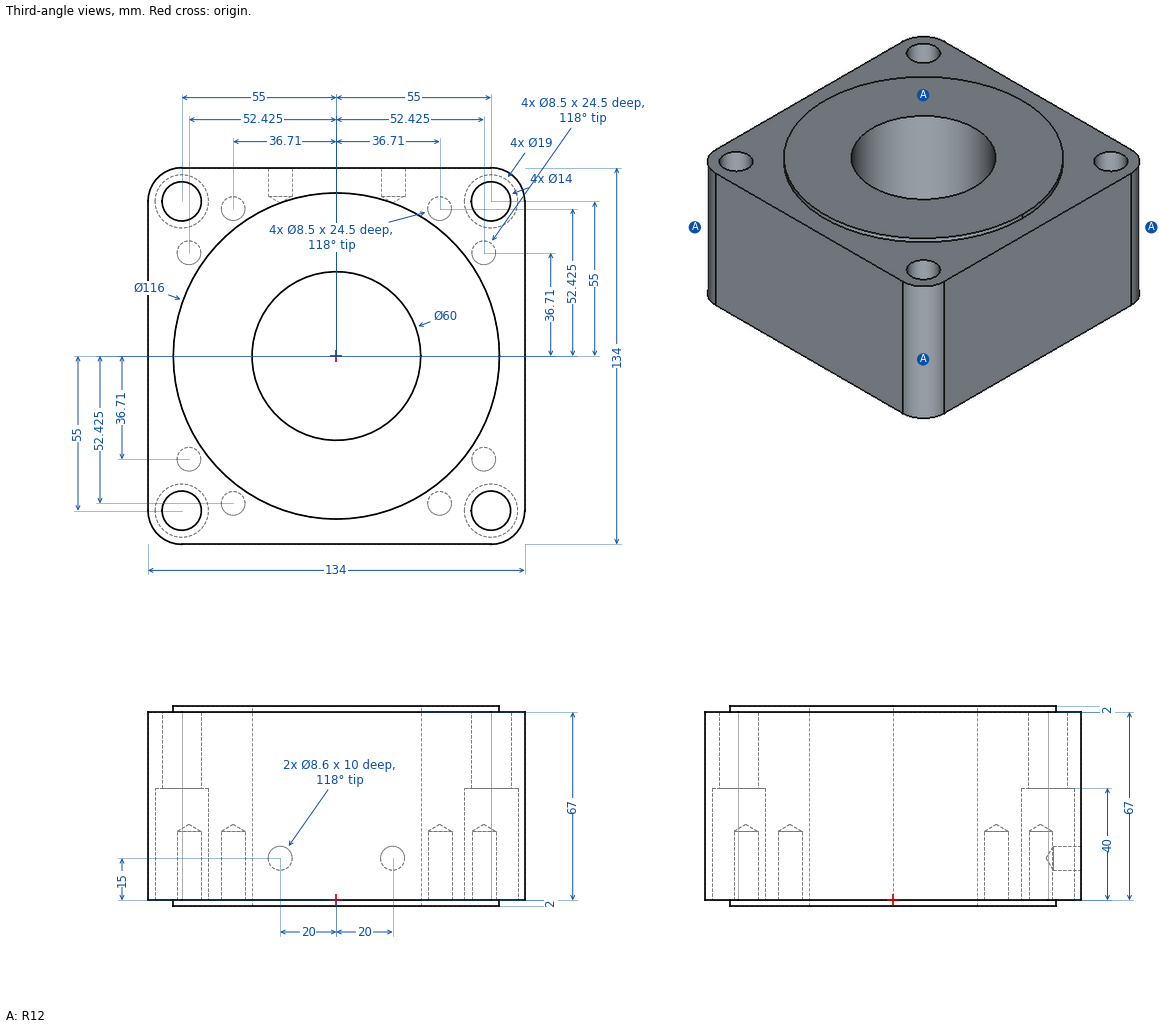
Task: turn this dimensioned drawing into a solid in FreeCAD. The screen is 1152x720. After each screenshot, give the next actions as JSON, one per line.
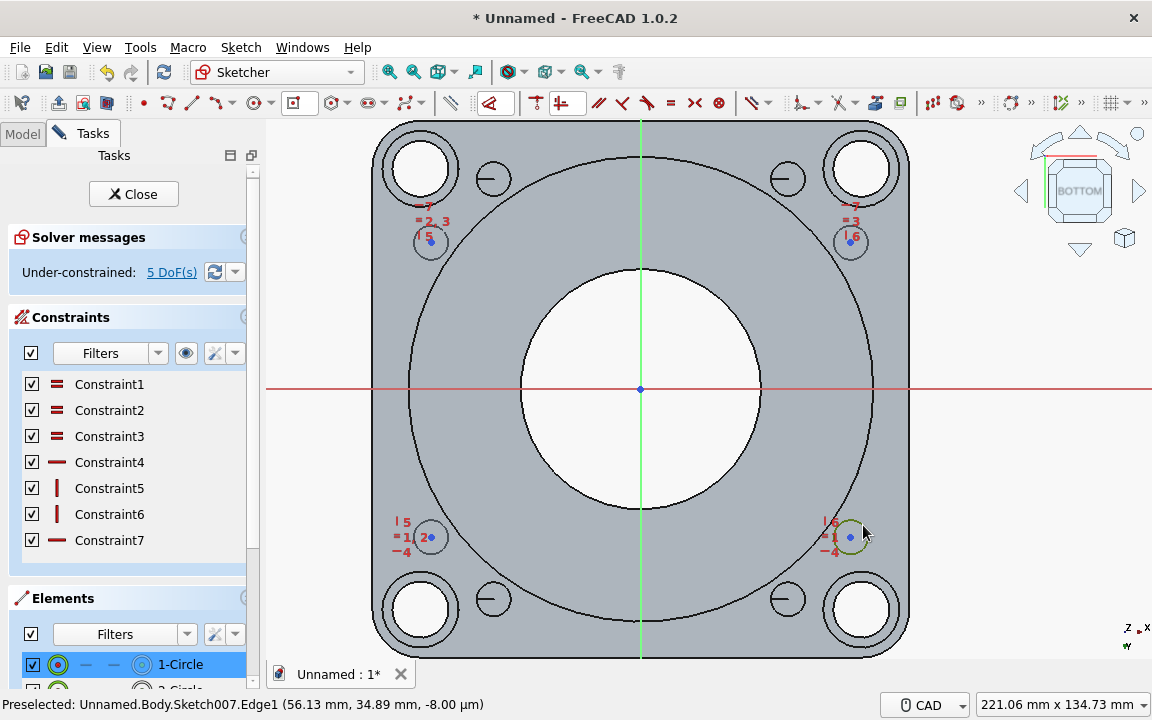
{"action": "left_click", "coordinate": [508, 104]}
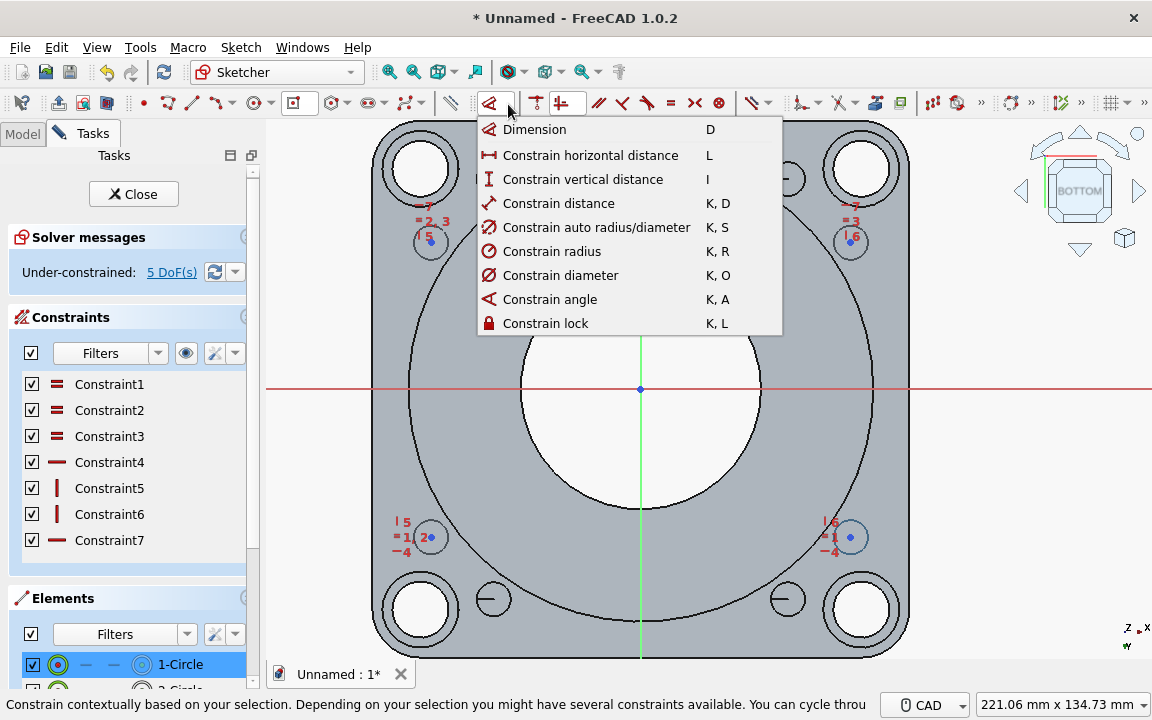
{"action": "left_click", "coordinate": [630, 275]}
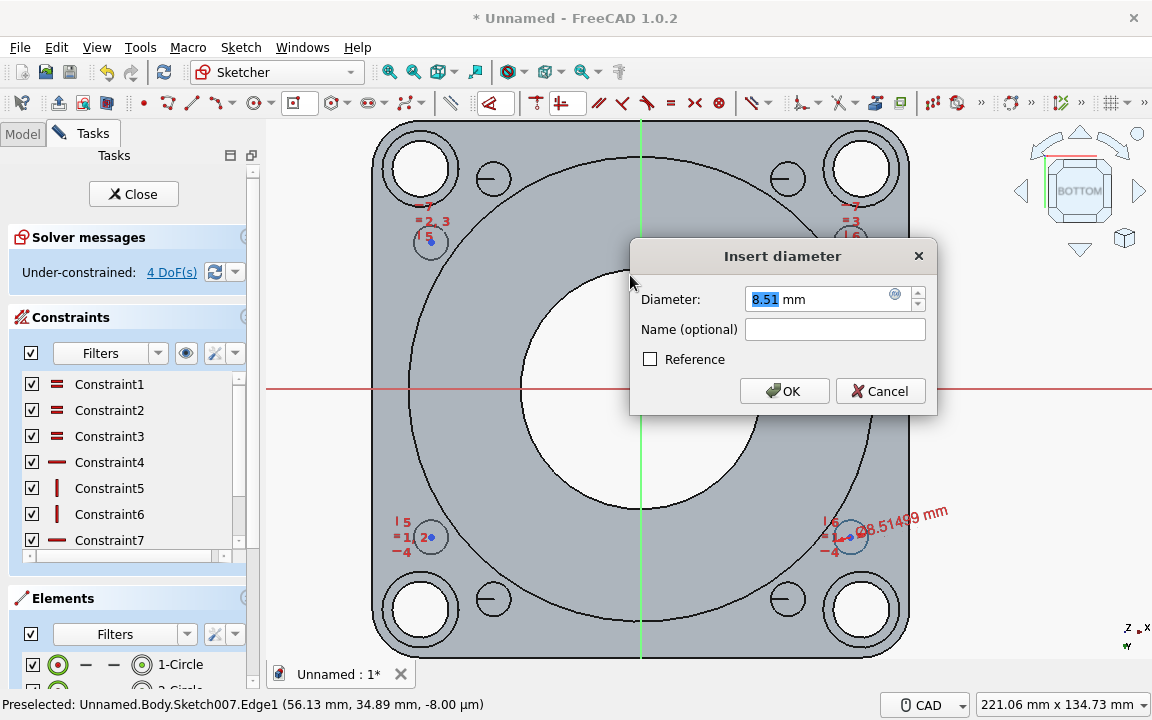
{"action": "type", "text": "8.5"}
{"action": "key", "text": "Return"}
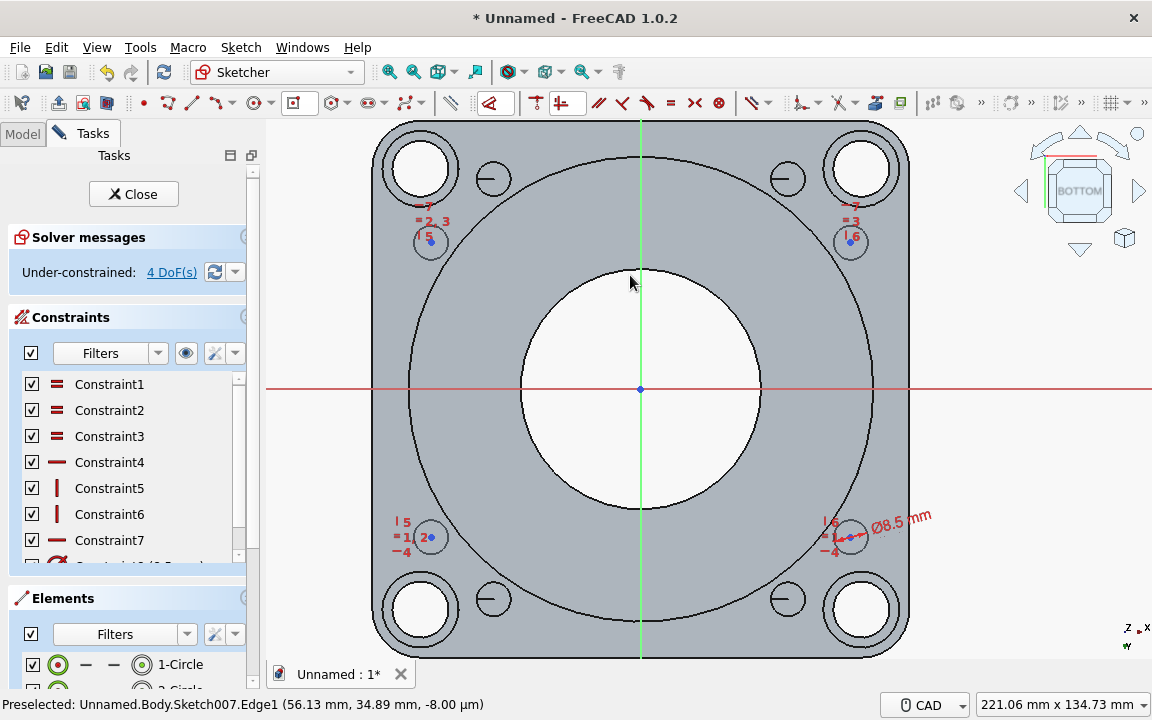
{"action": "left_click", "coordinate": [851, 537]}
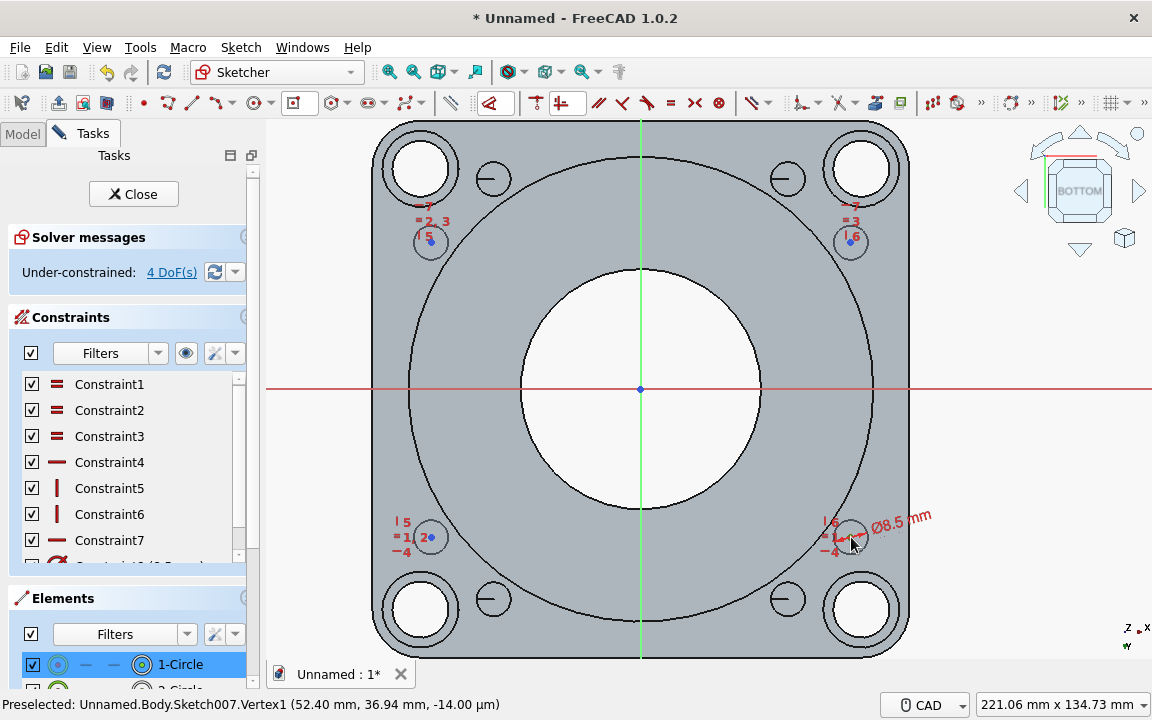
{"action": "left_click", "coordinate": [508, 104]}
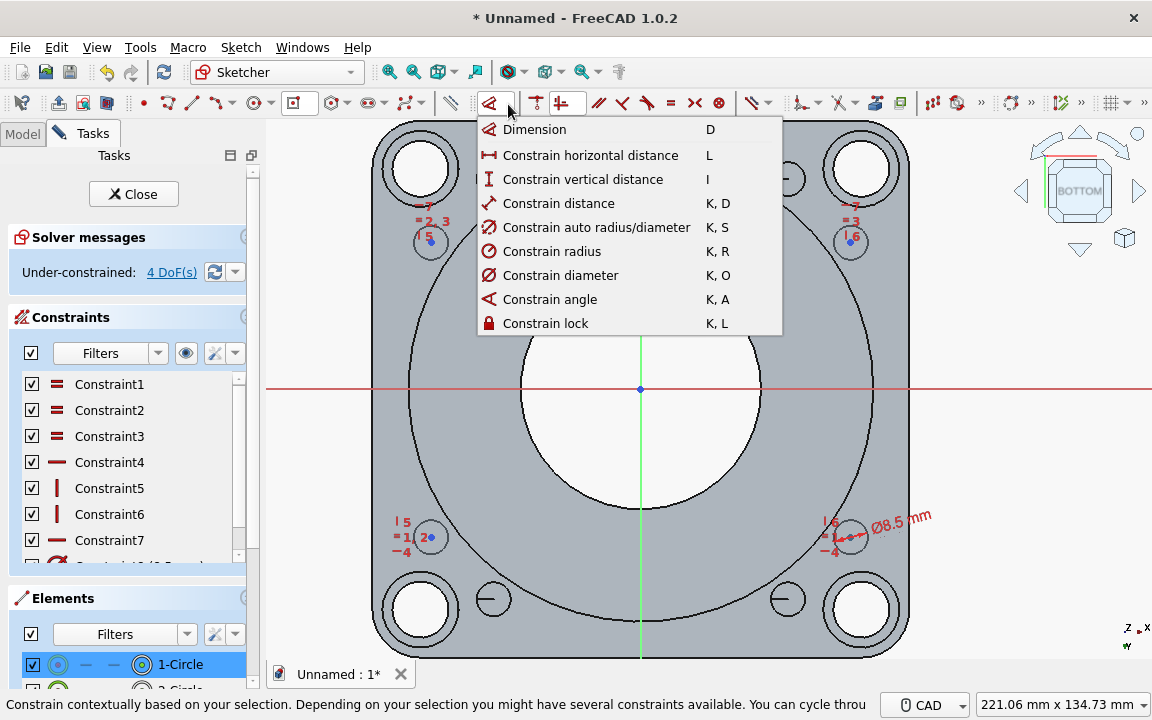
{"action": "left_click", "coordinate": [630, 179]}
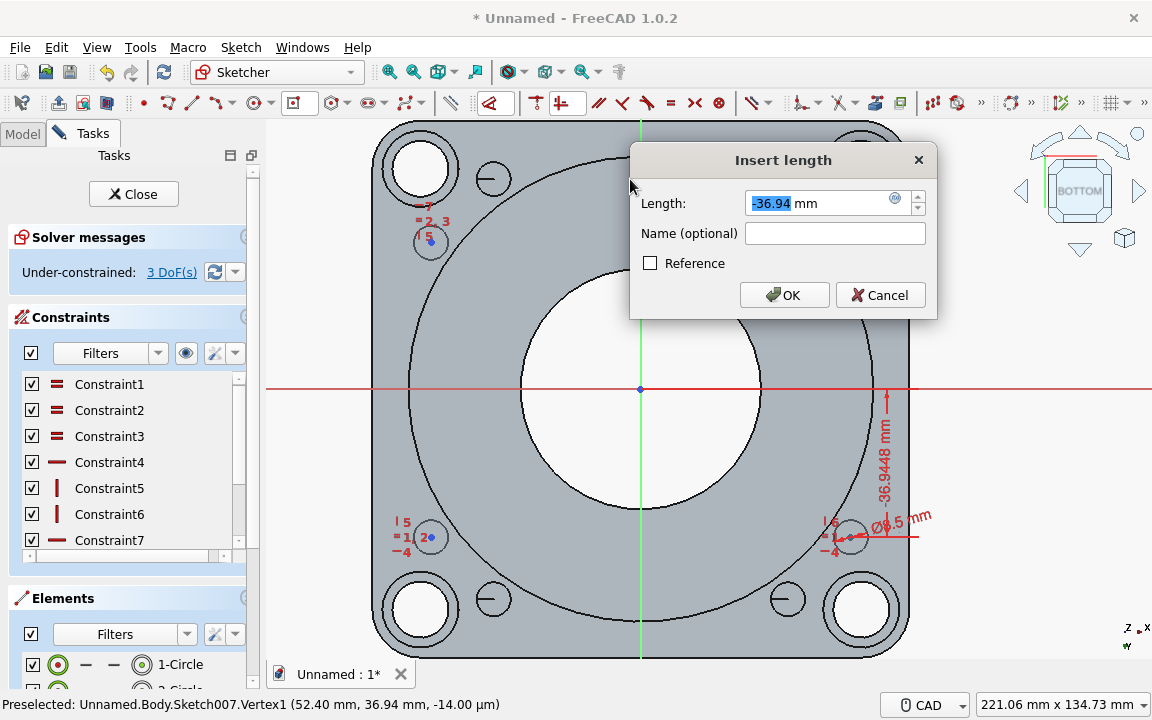
{"action": "type", "text": "-36.71"}
{"action": "key", "text": "Return"}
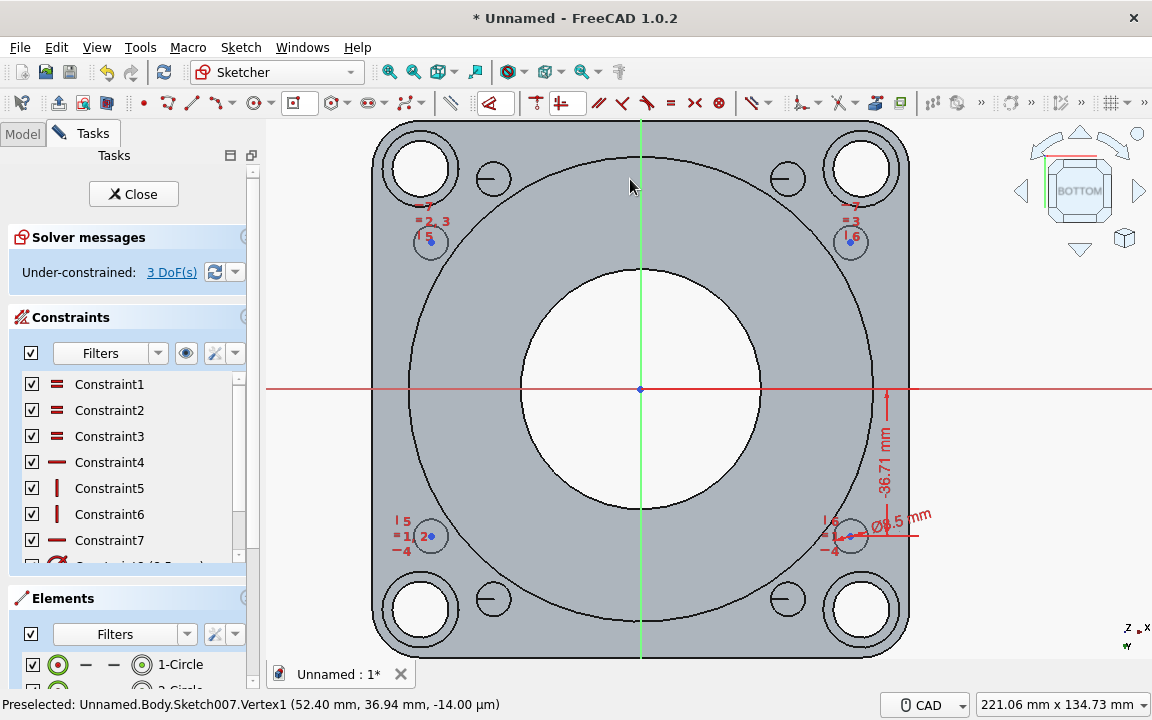
{"action": "left_click", "coordinate": [431, 243]}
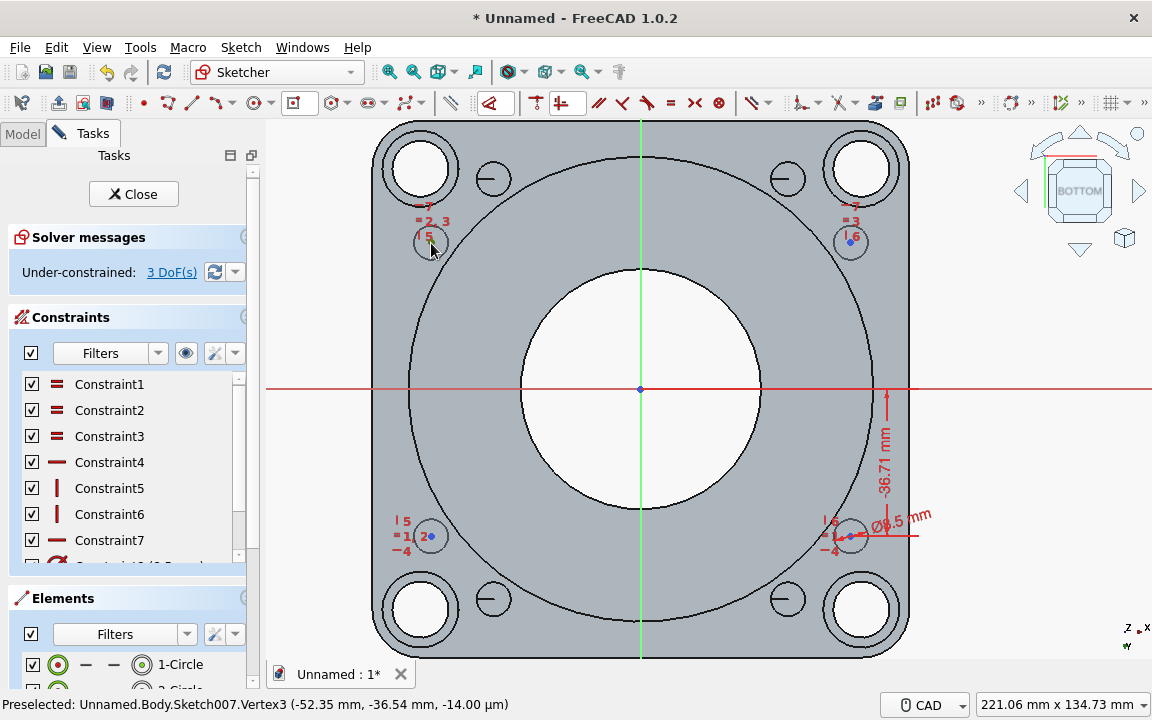
{"action": "left_click", "coordinate": [508, 104]}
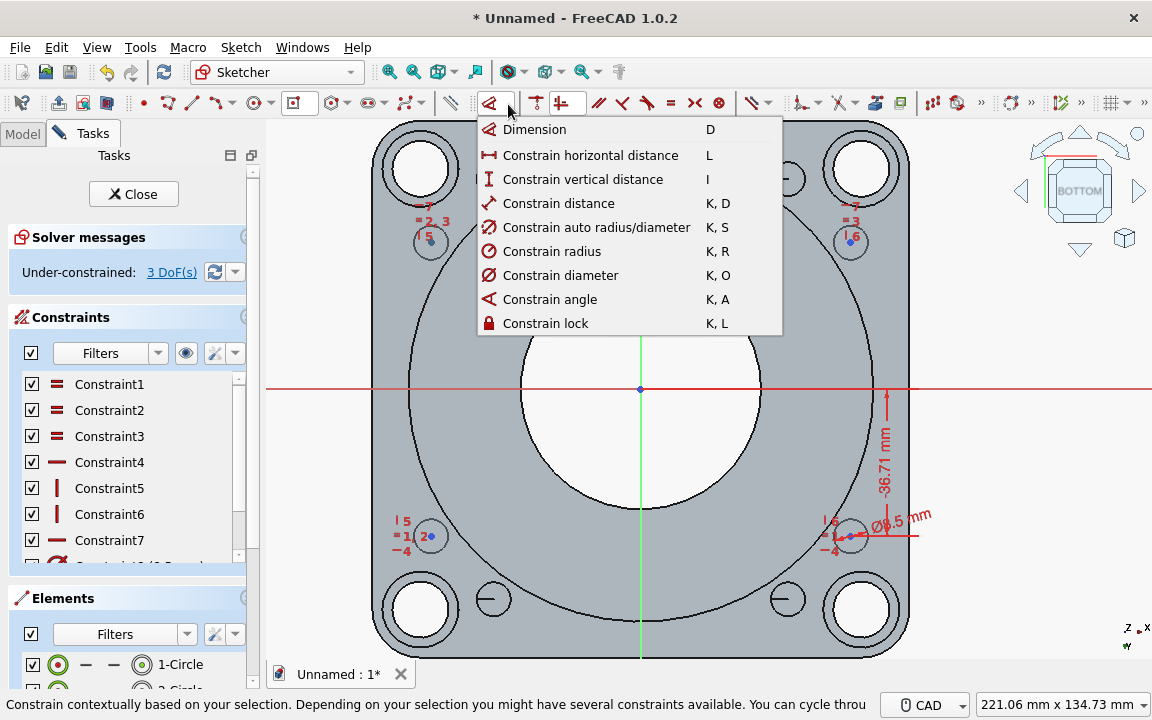
{"action": "left_click", "coordinate": [630, 179]}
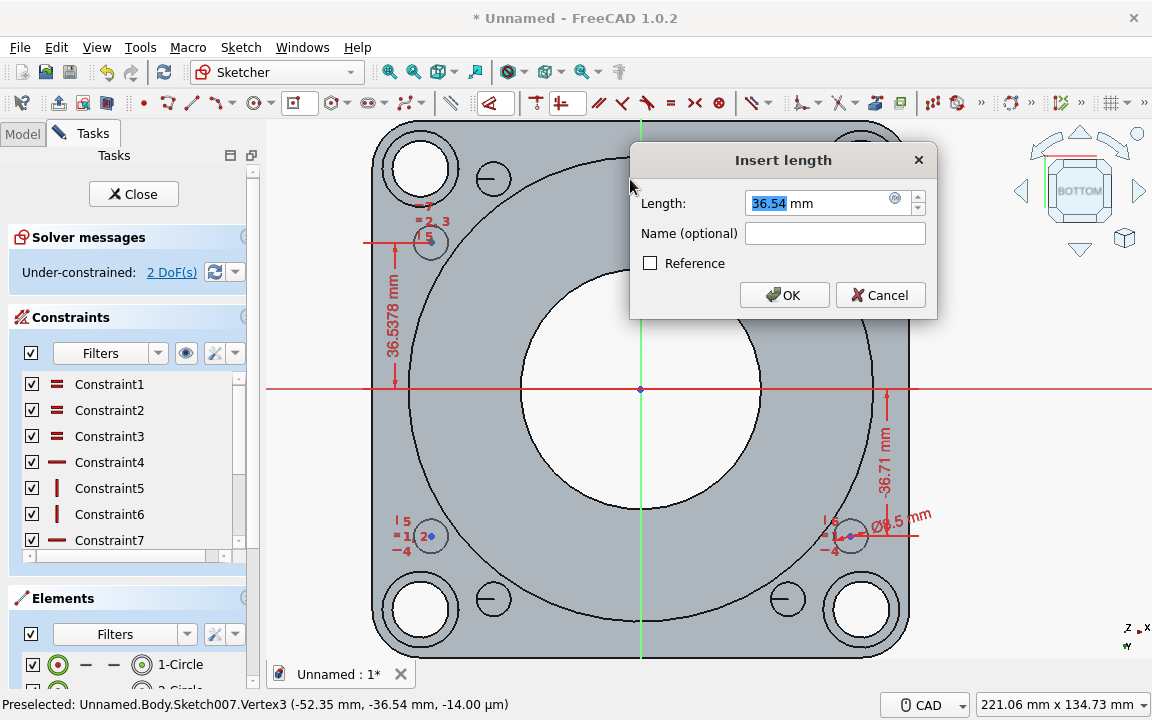
{"action": "type", "text": "36.71"}
{"action": "key", "text": "Return"}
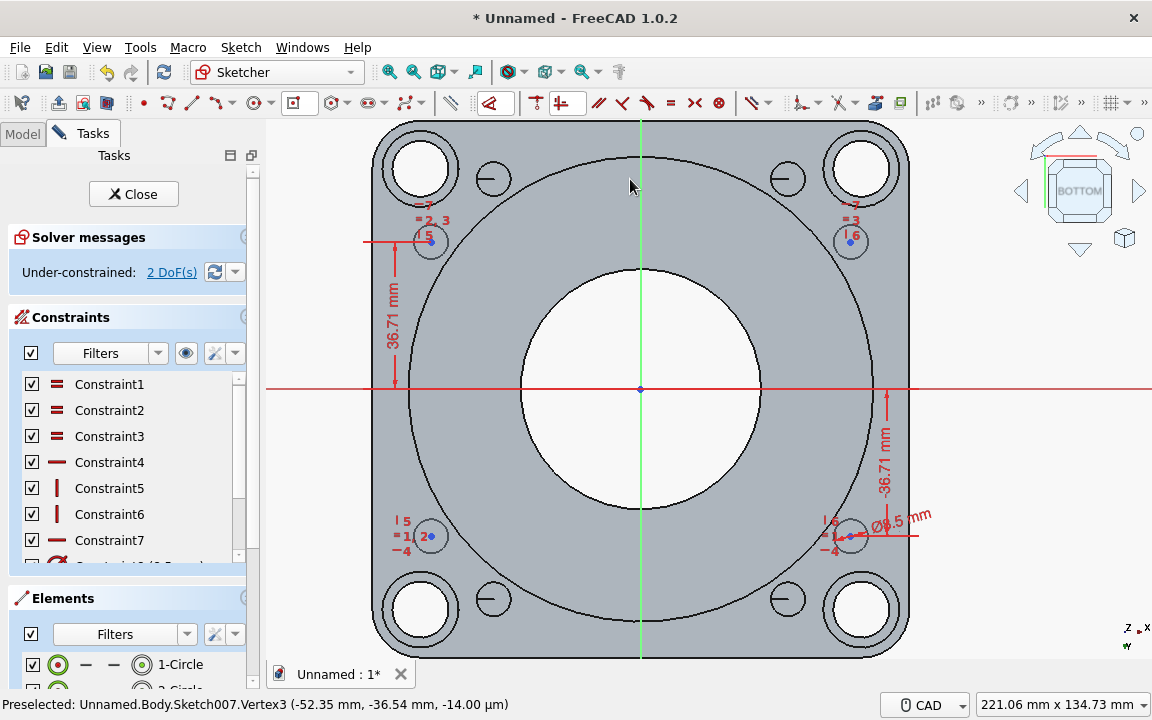
{"action": "left_click", "coordinate": [851, 536]}